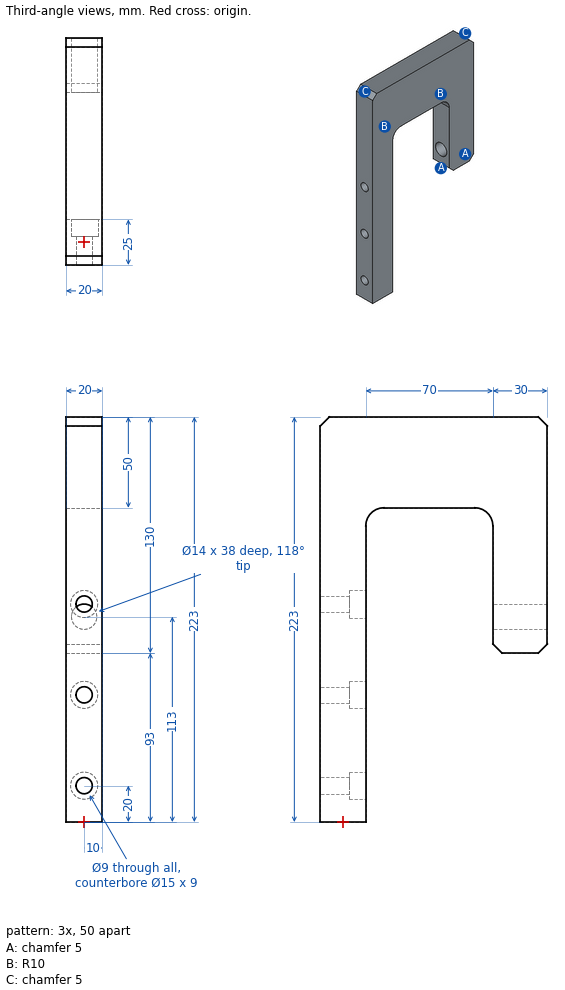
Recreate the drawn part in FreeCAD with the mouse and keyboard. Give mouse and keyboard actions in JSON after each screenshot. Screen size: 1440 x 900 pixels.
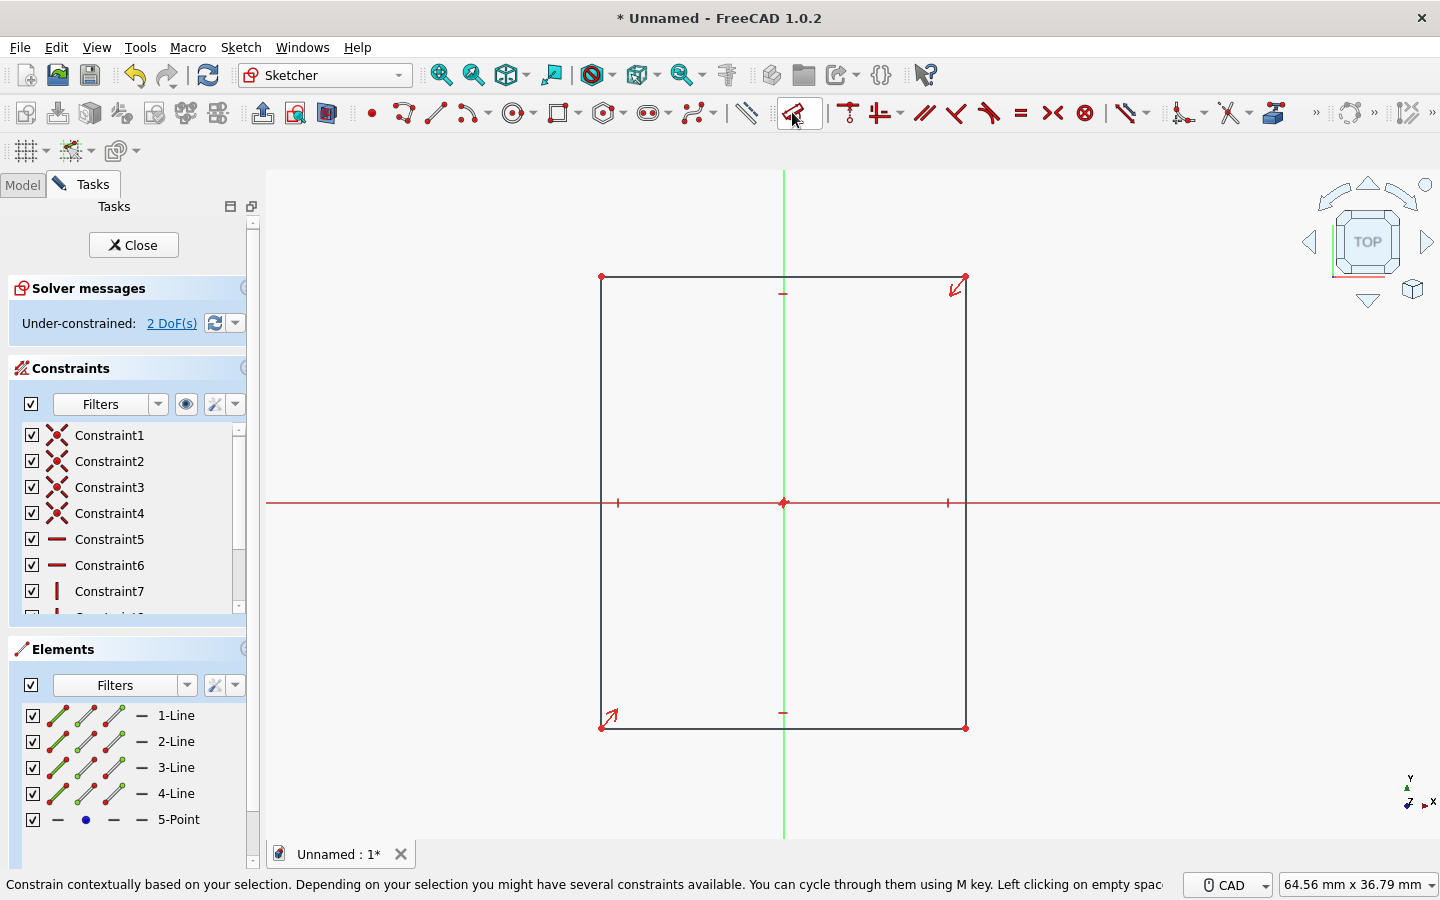
{"action": "left_click", "coordinate": [711, 729]}
{"action": "left_click", "coordinate": [700, 763]}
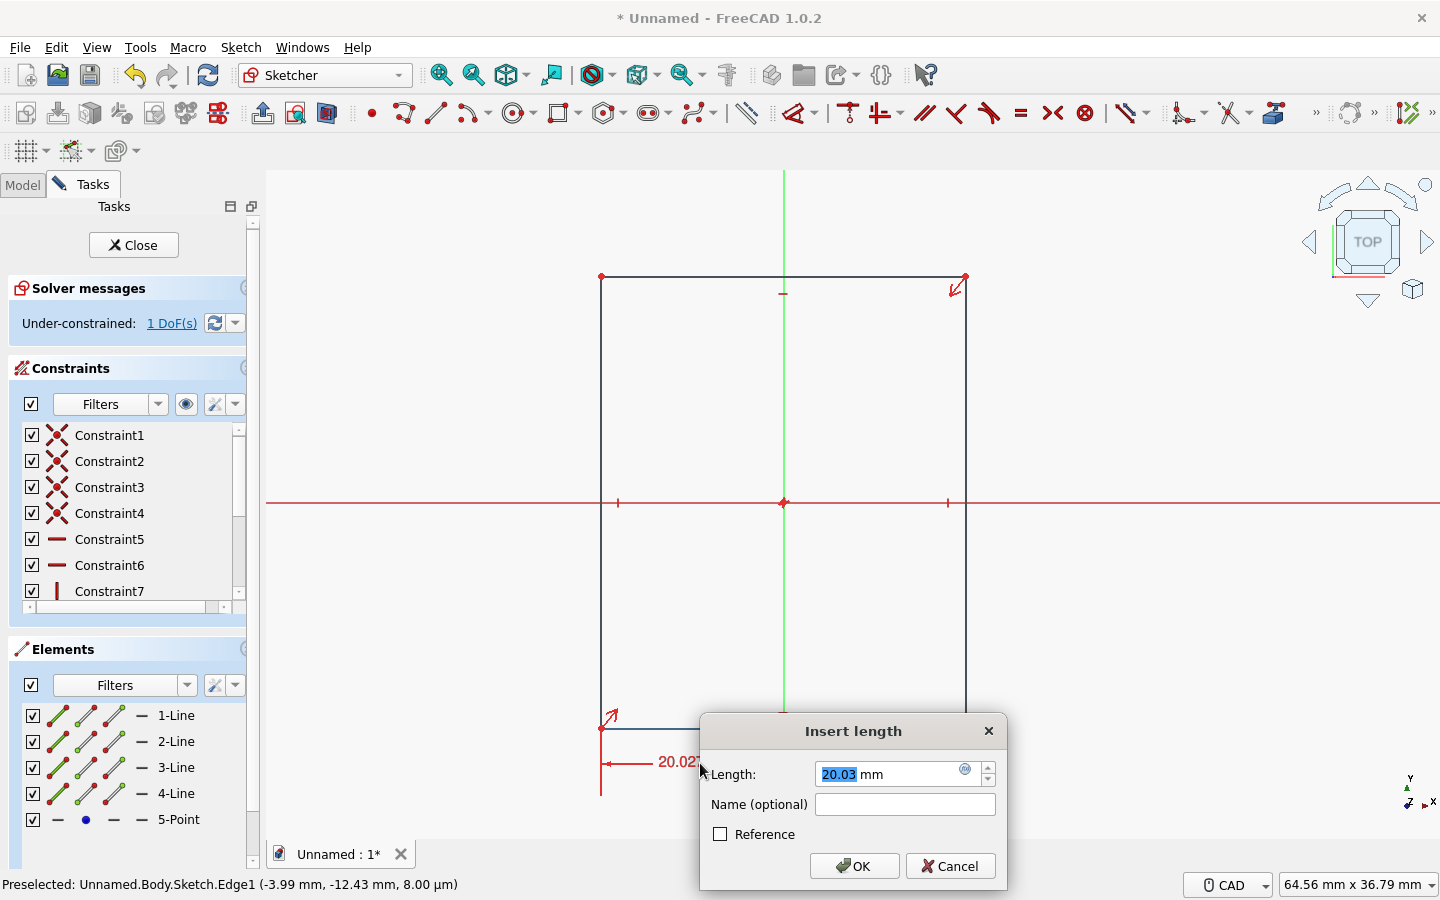
{"action": "type", "text": "20"}
{"action": "key", "text": "Return"}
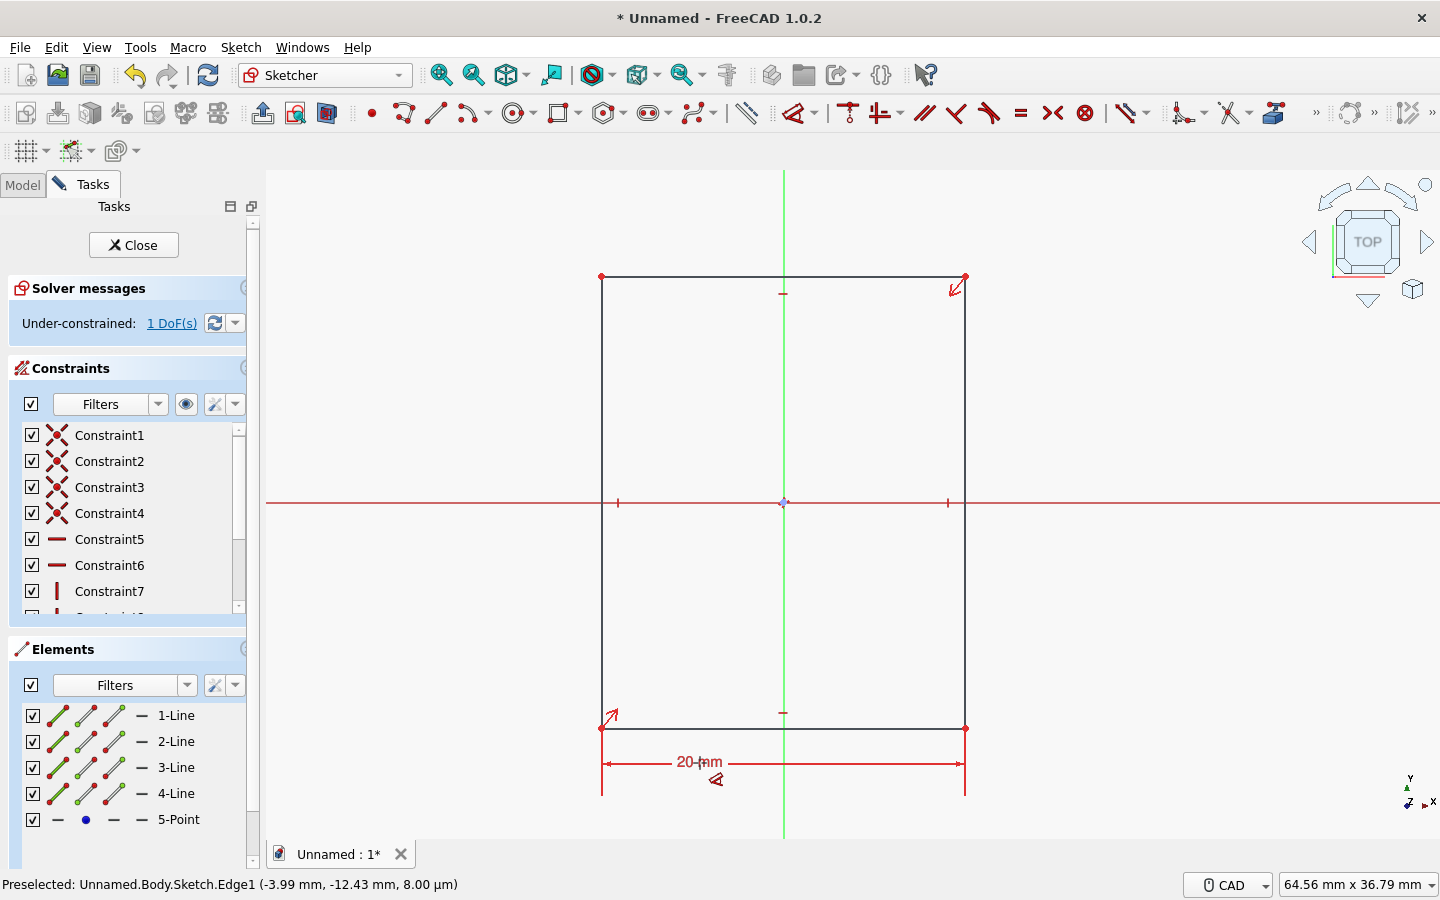
{"action": "left_click", "coordinate": [965, 593]}
{"action": "left_click", "coordinate": [999, 399]}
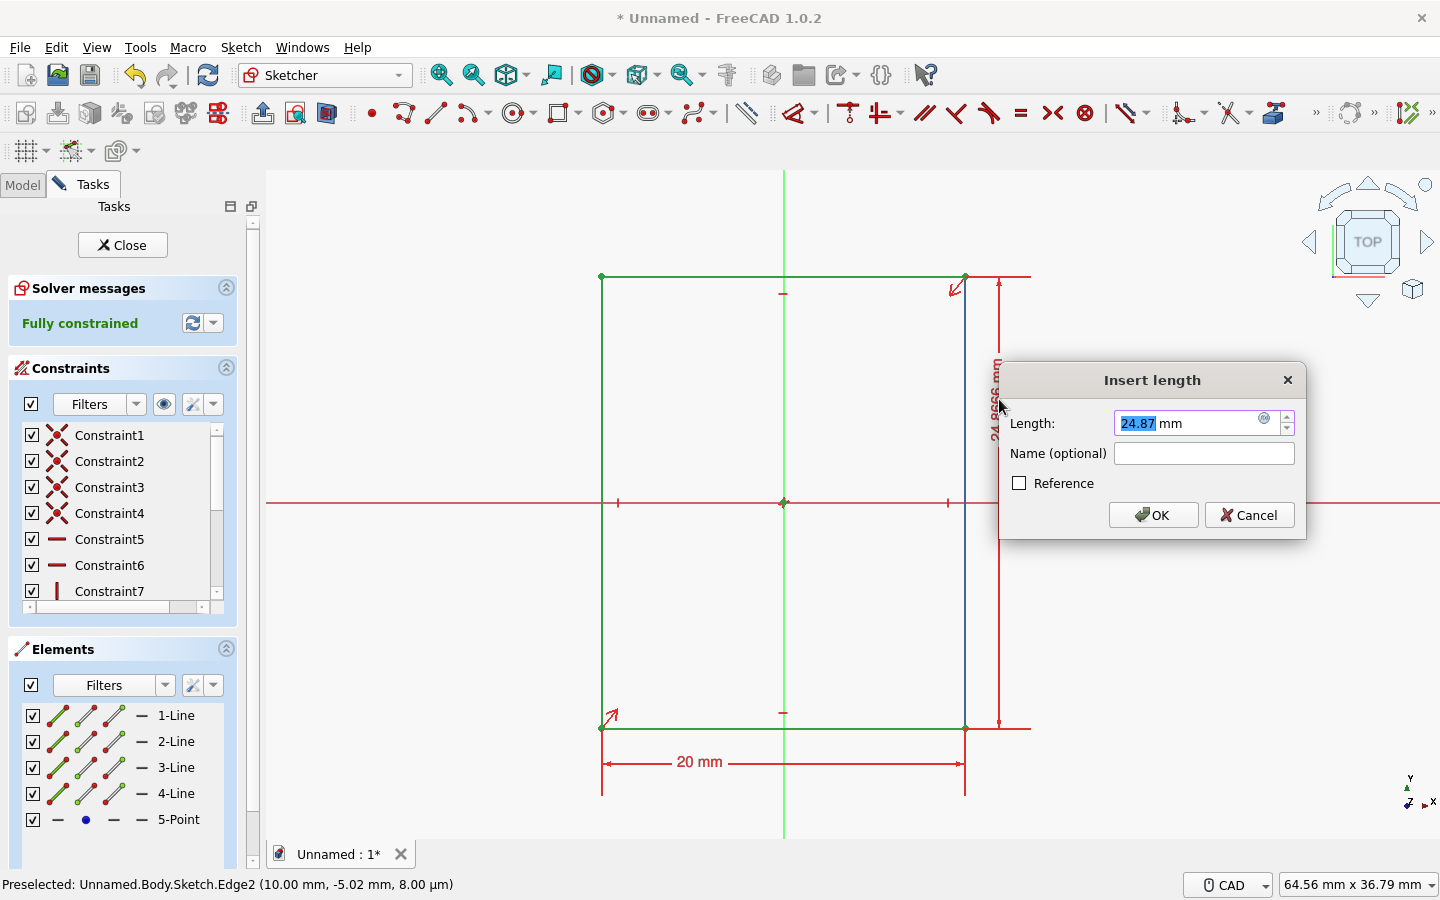
{"action": "type", "text": "25"}
{"action": "key", "text": "Return"}
{"action": "key", "text": "Escape"}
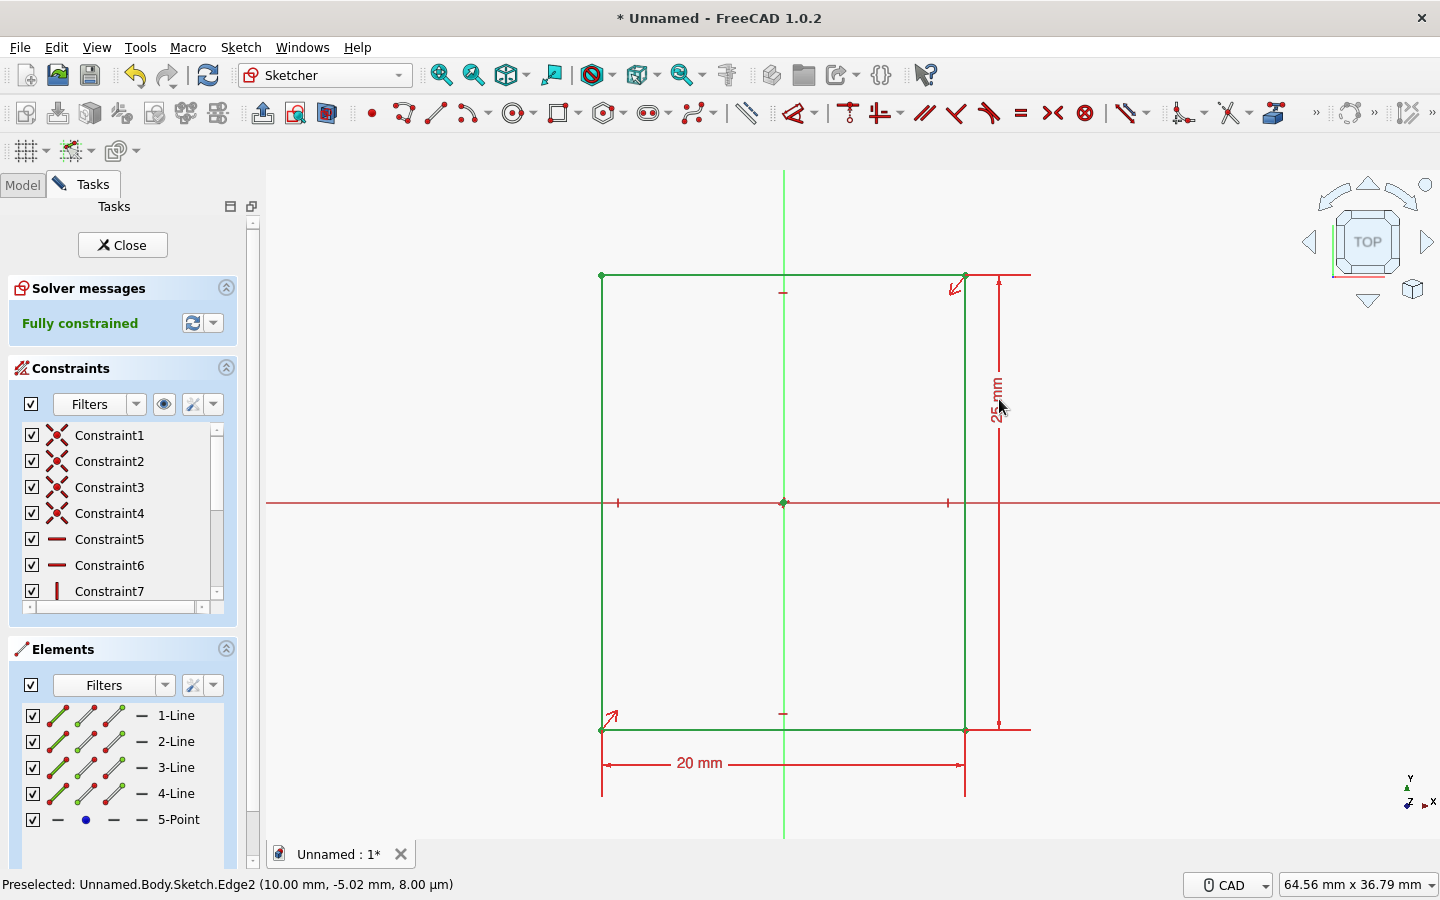
{"action": "left_click", "coordinate": [123, 245]}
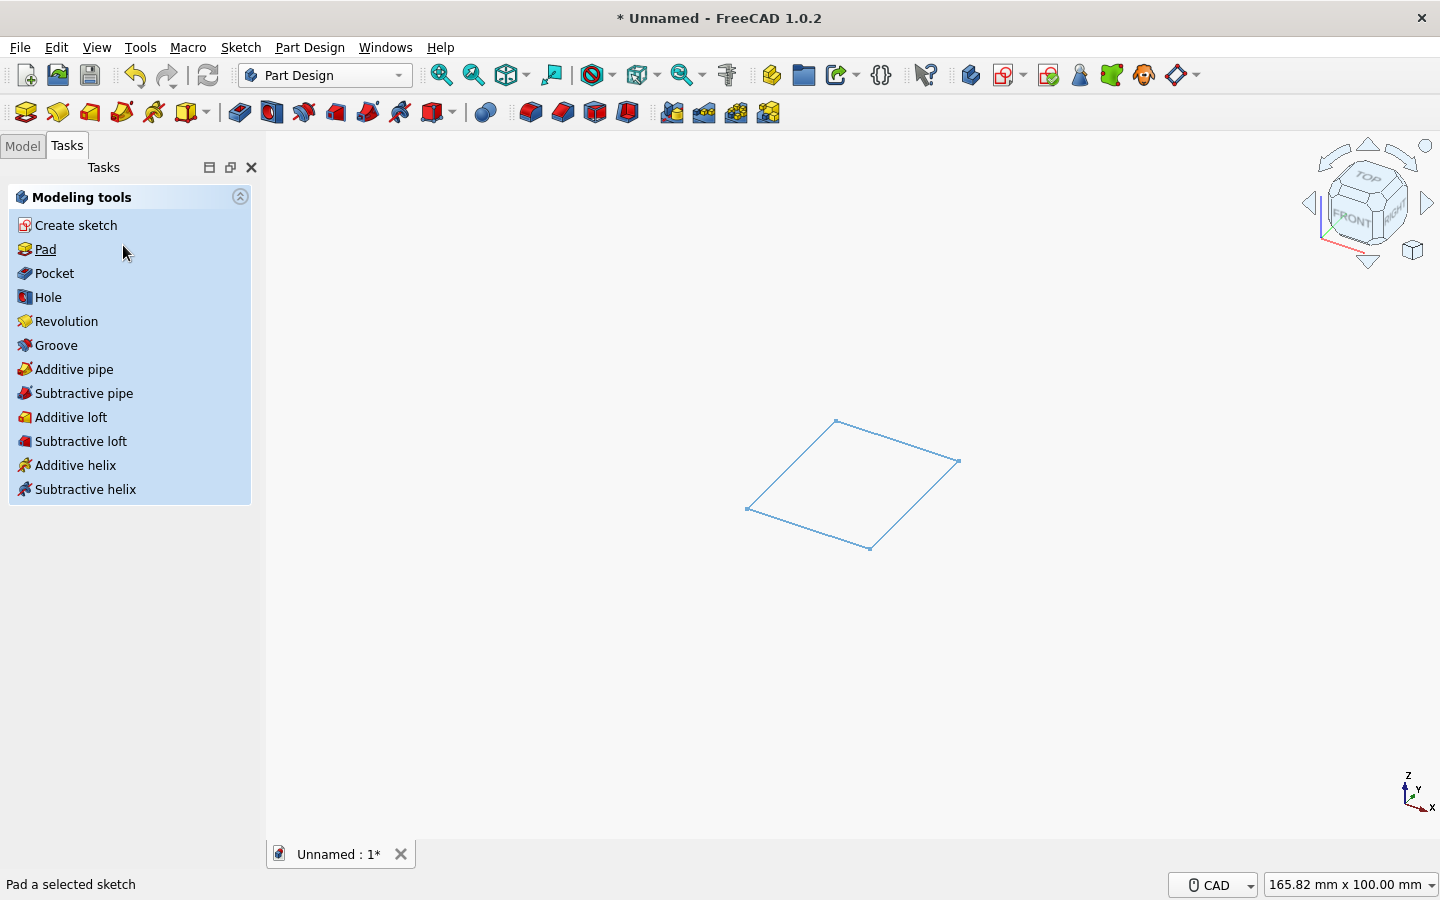
{"action": "left_click", "coordinate": [26, 112]}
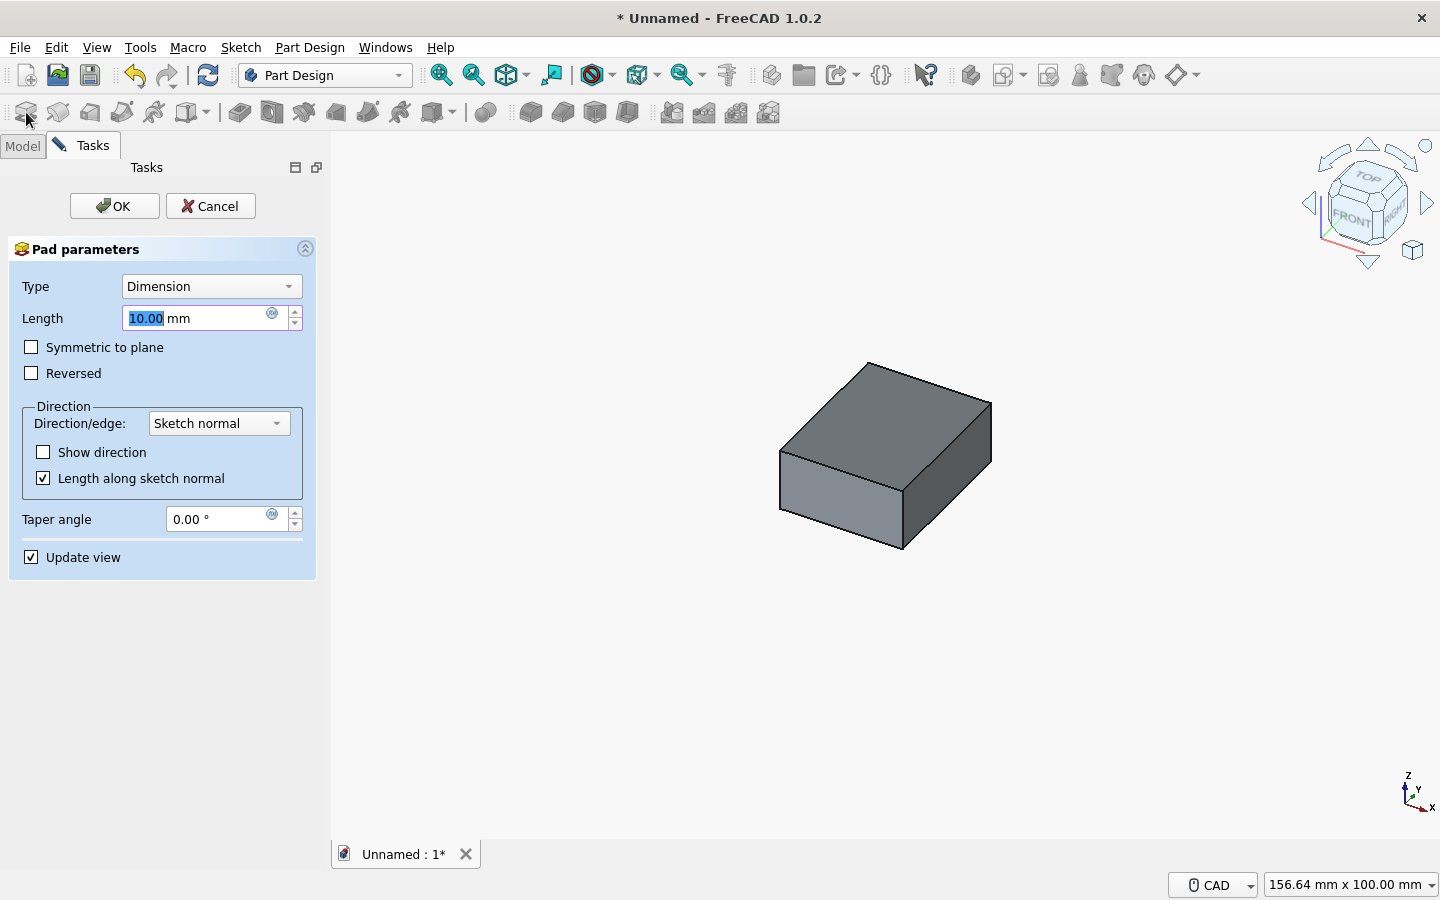
{"action": "type", "text": "223"}
{"action": "key", "text": "Tab"}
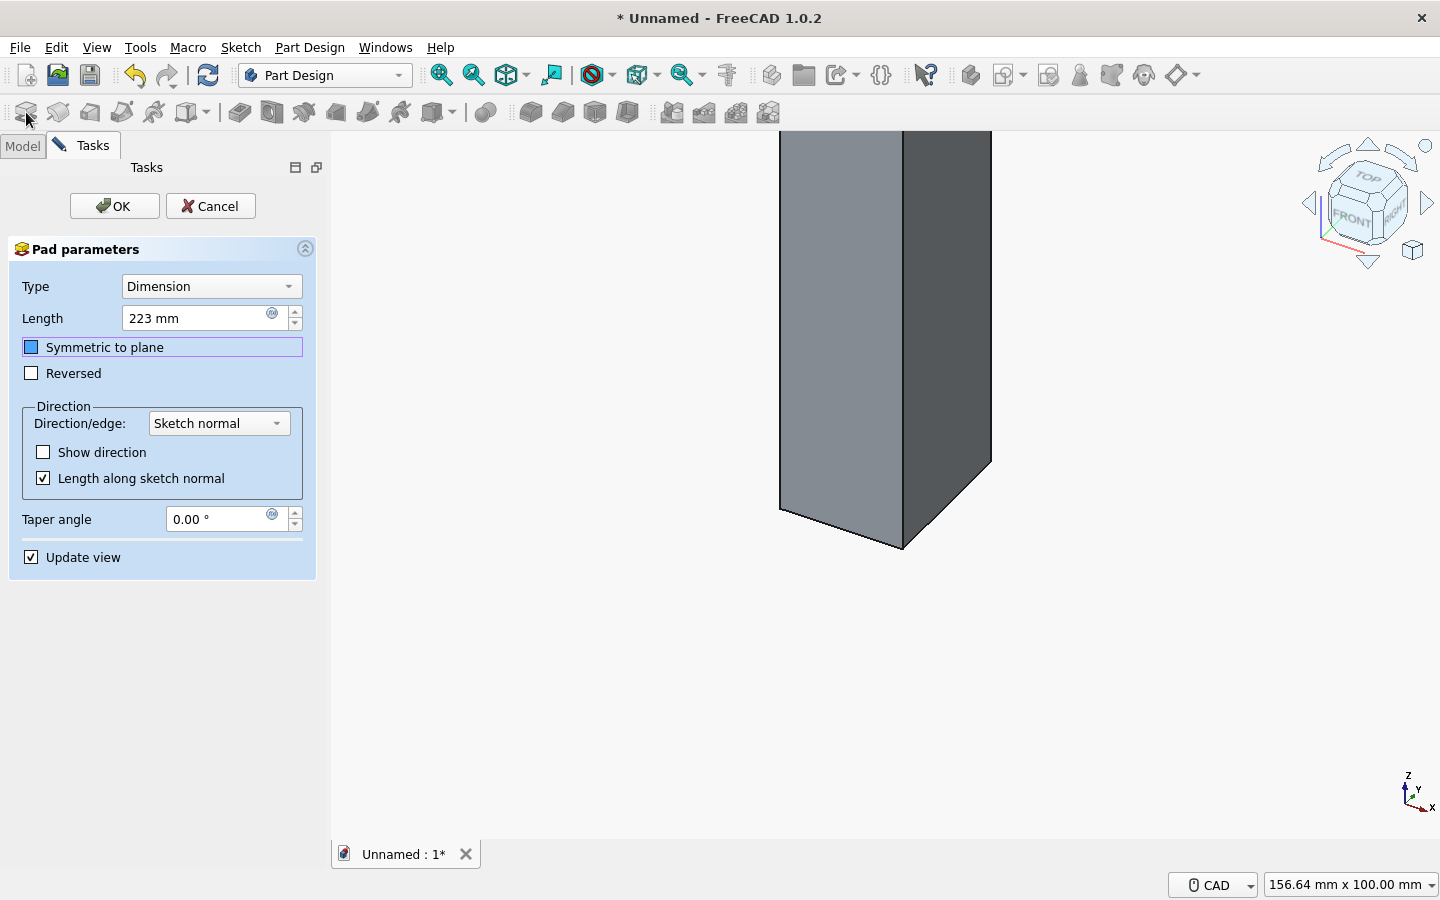
{"action": "left_click", "coordinate": [115, 206]}